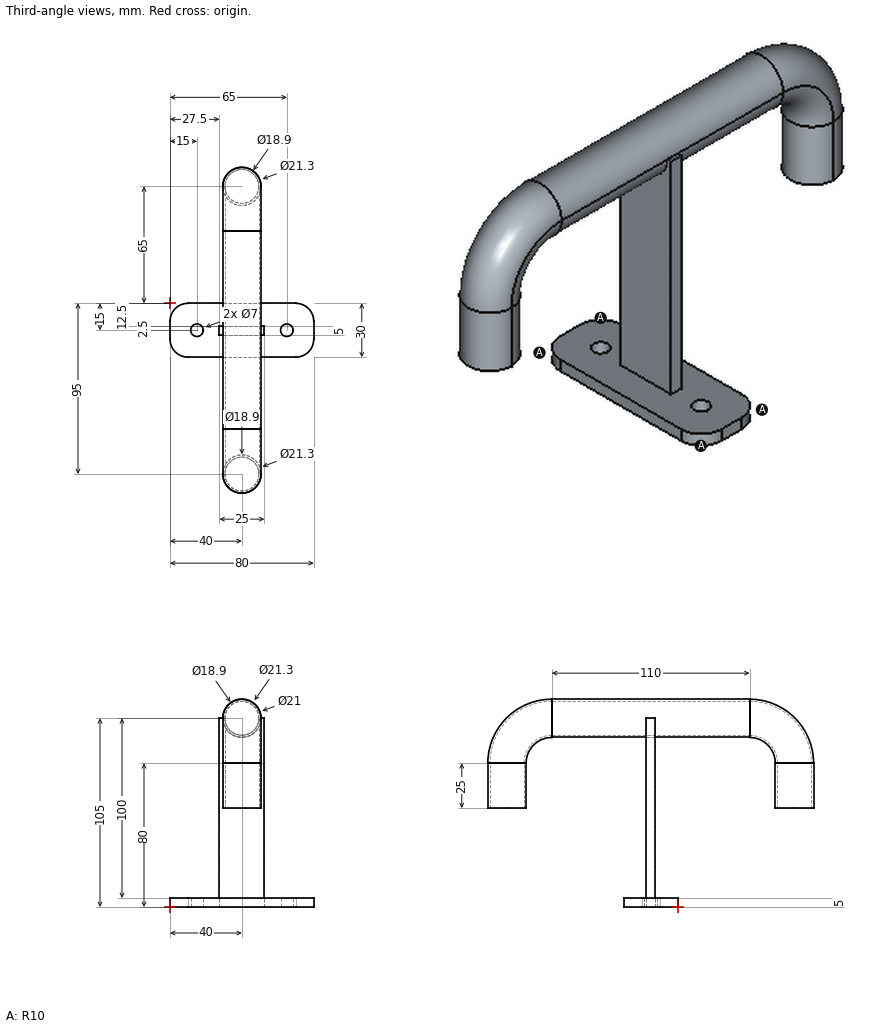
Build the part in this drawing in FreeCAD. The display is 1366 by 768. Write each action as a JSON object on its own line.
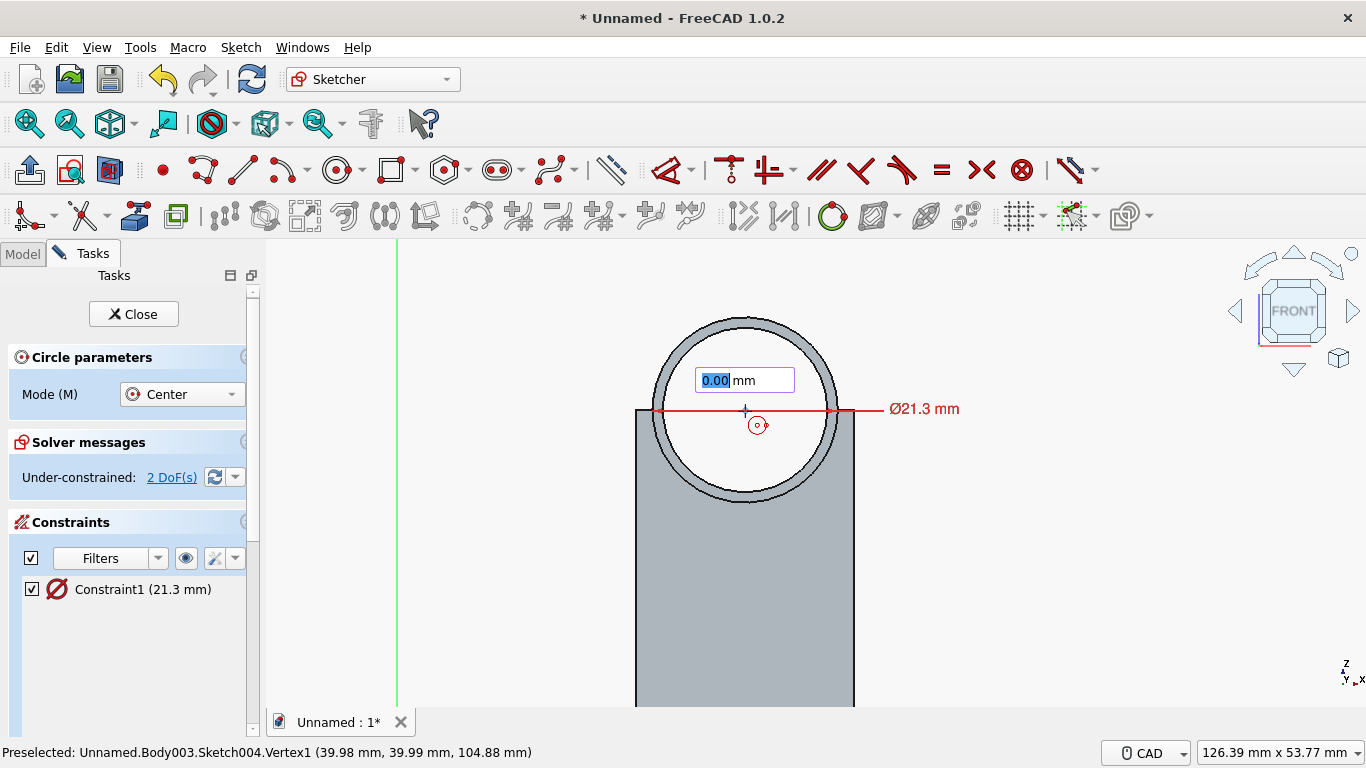
{"action": "scroll", "coordinate": [803, 468], "scroll_direction": "up", "scroll_amount": 3}
{"action": "mouse_move", "coordinate": [803, 468]}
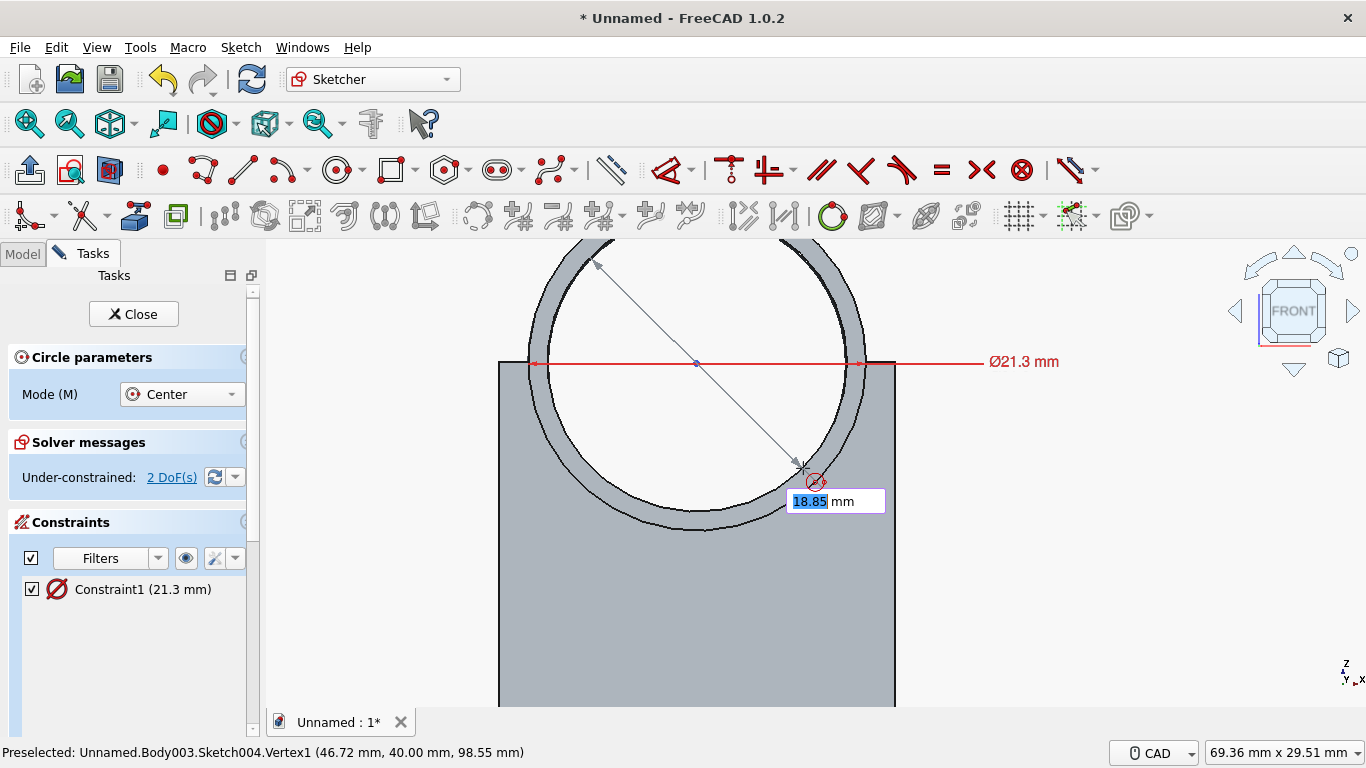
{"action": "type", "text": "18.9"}
{"action": "key", "text": "Return"}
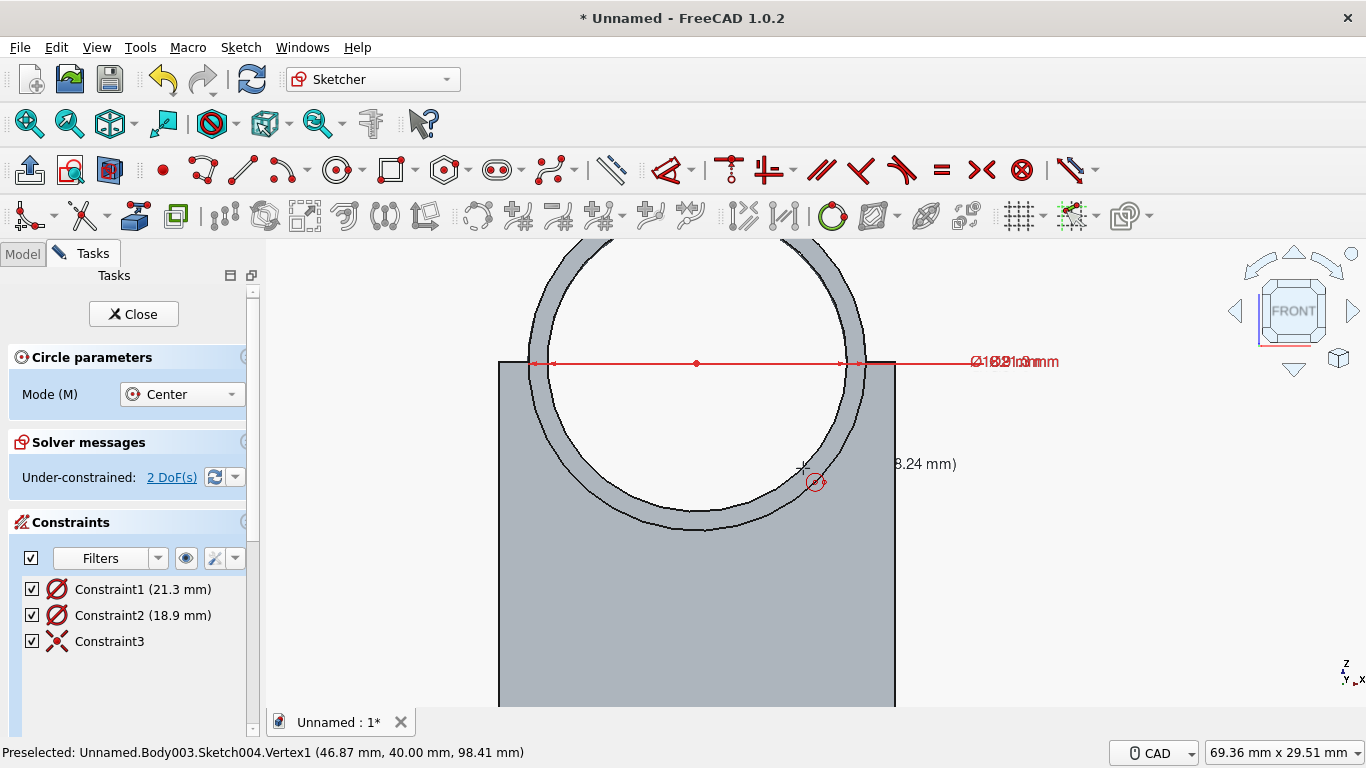
{"action": "left_click", "coordinate": [244, 170]}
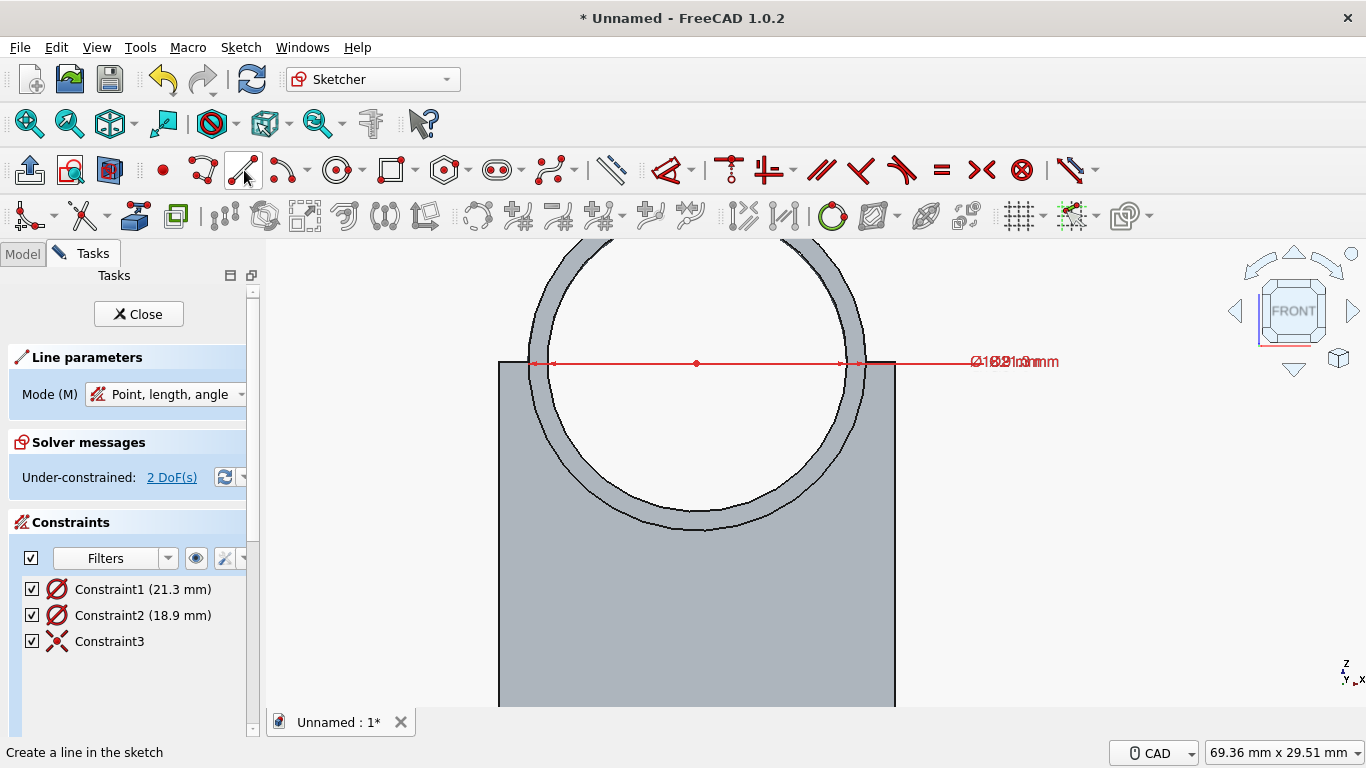
{"action": "scroll", "coordinate": [809, 470], "scroll_direction": "down", "scroll_amount": 3}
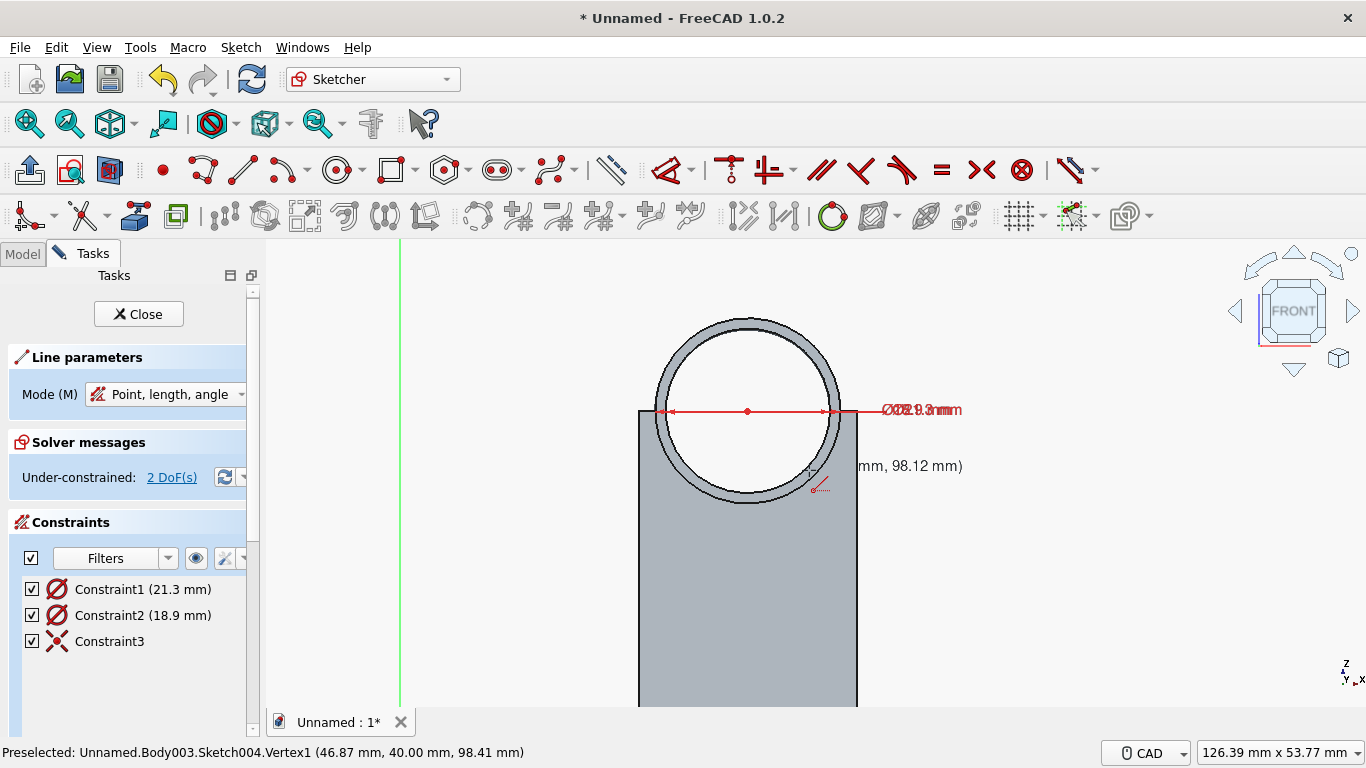
{"action": "left_click", "coordinate": [859, 628]}
{"action": "left_click", "coordinate": [637, 628]}
{"action": "key", "text": "Escape"}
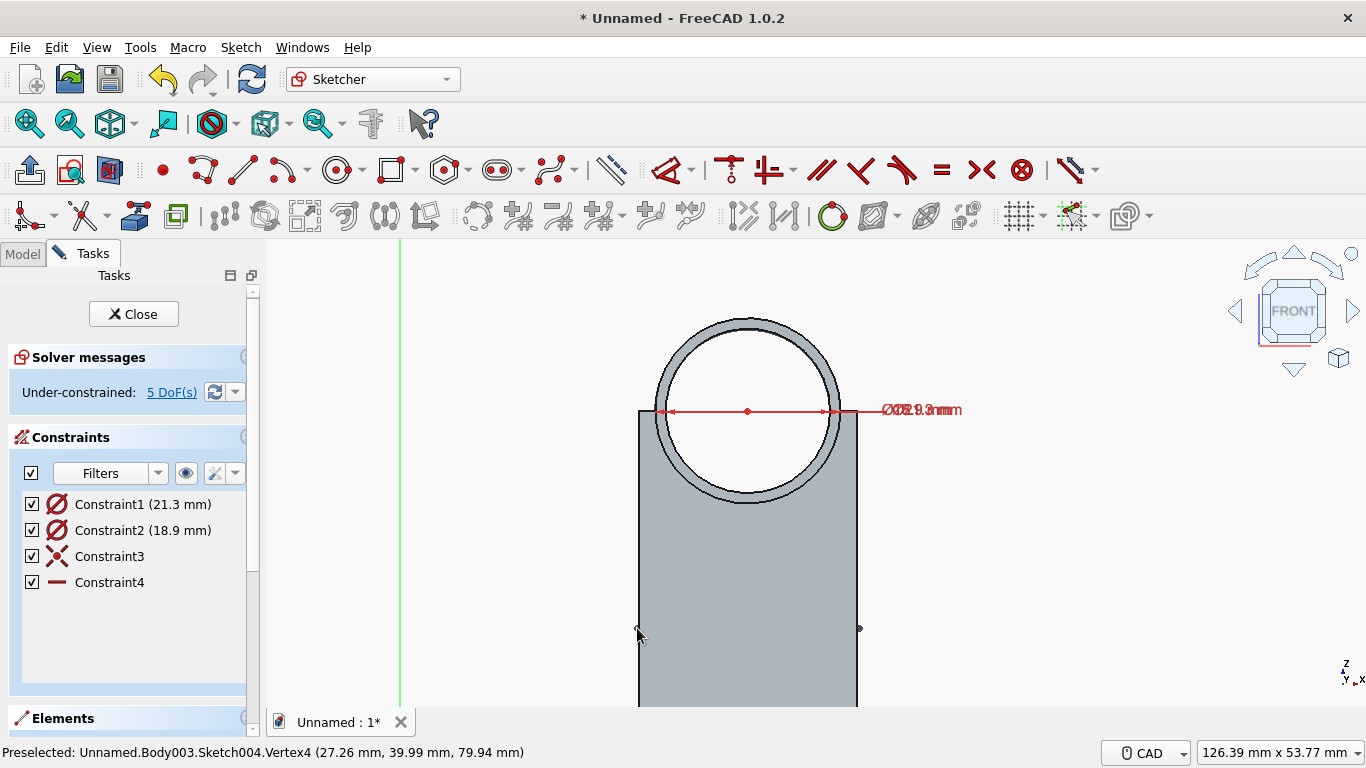
{"action": "left_click", "coordinate": [792, 629]}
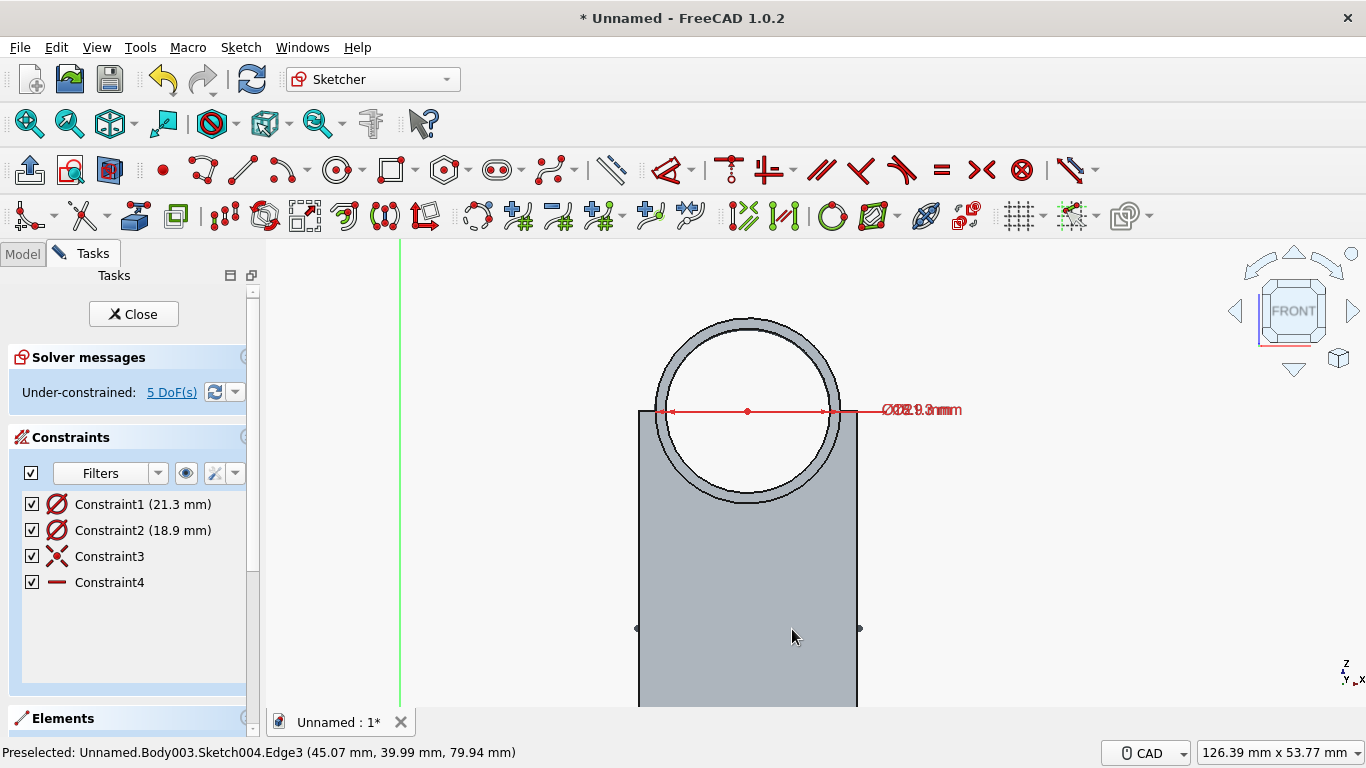
{"action": "left_click", "coordinate": [612, 170]}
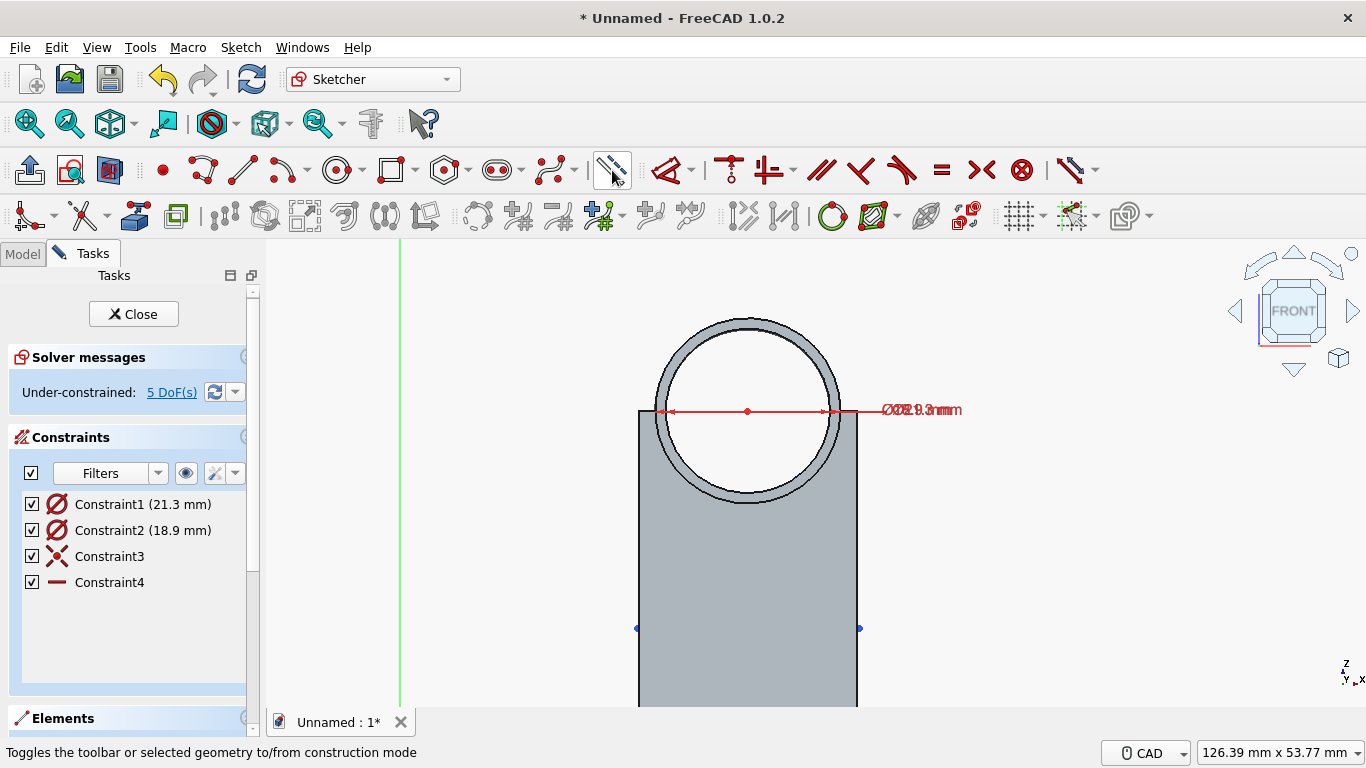
{"action": "left_click", "coordinate": [666, 170]}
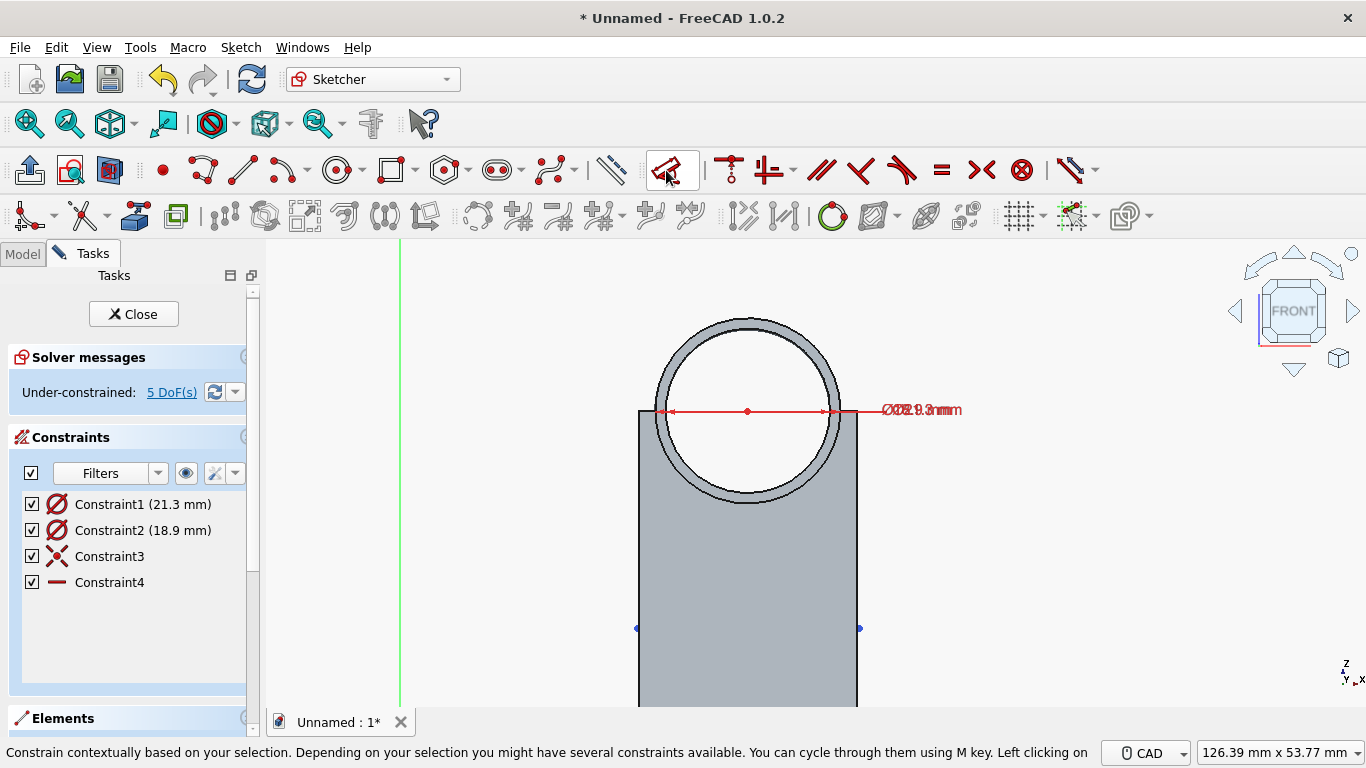
{"action": "left_click", "coordinate": [748, 412]}
{"action": "left_click", "coordinate": [574, 378]}